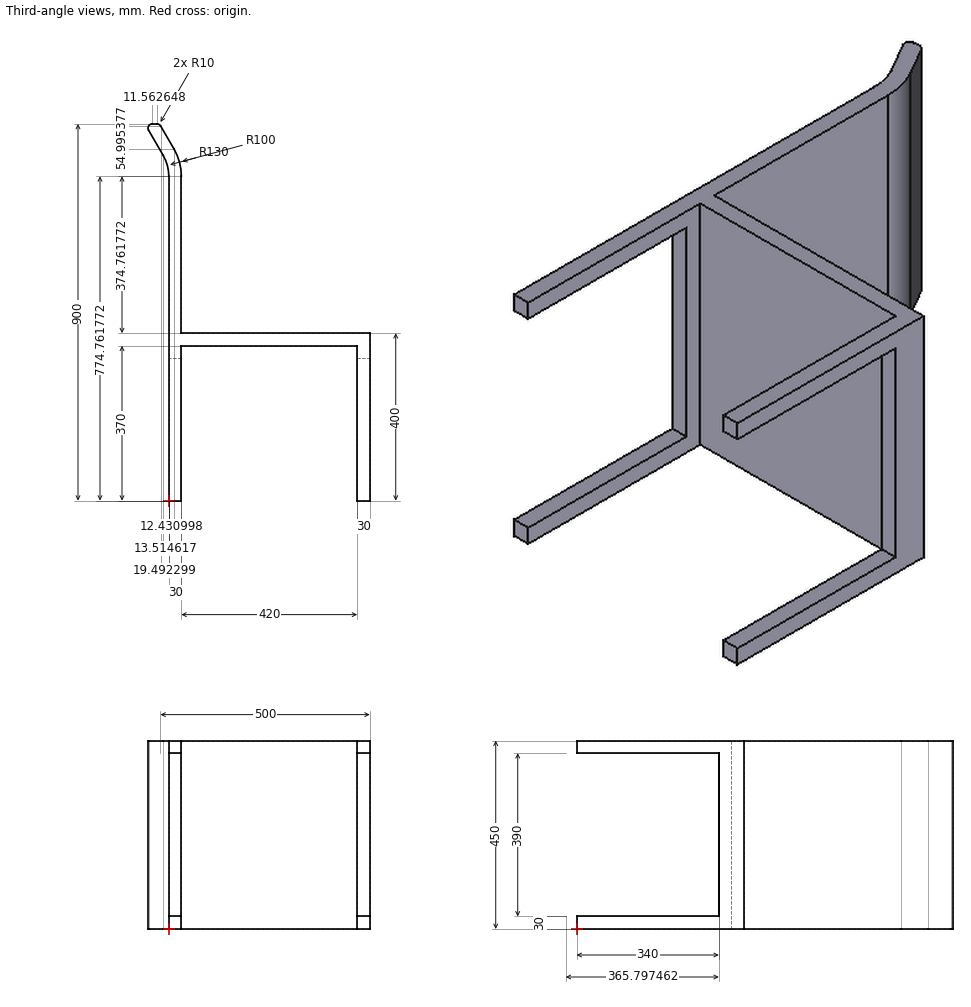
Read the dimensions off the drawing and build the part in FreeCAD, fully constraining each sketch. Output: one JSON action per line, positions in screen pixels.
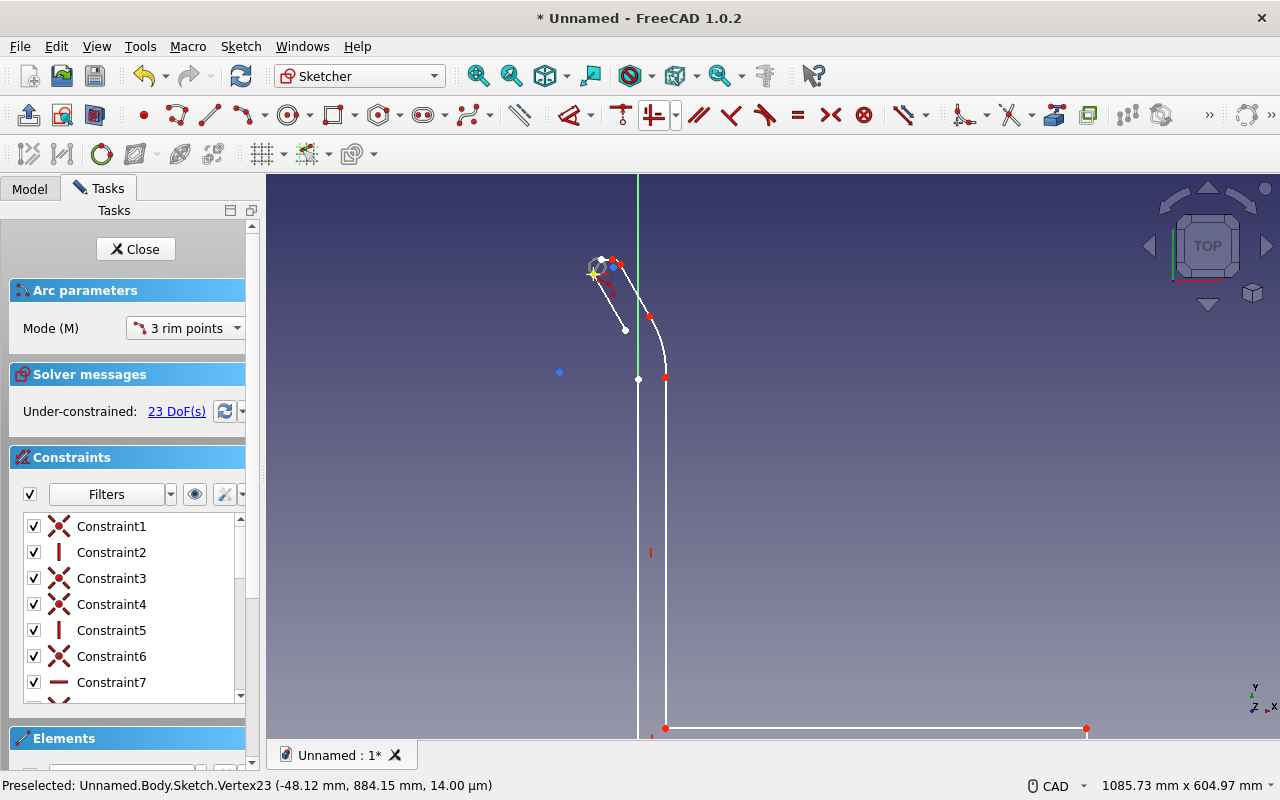
{"action": "scroll", "coordinate": [593, 264], "scroll_direction": "up", "scroll_amount": 7}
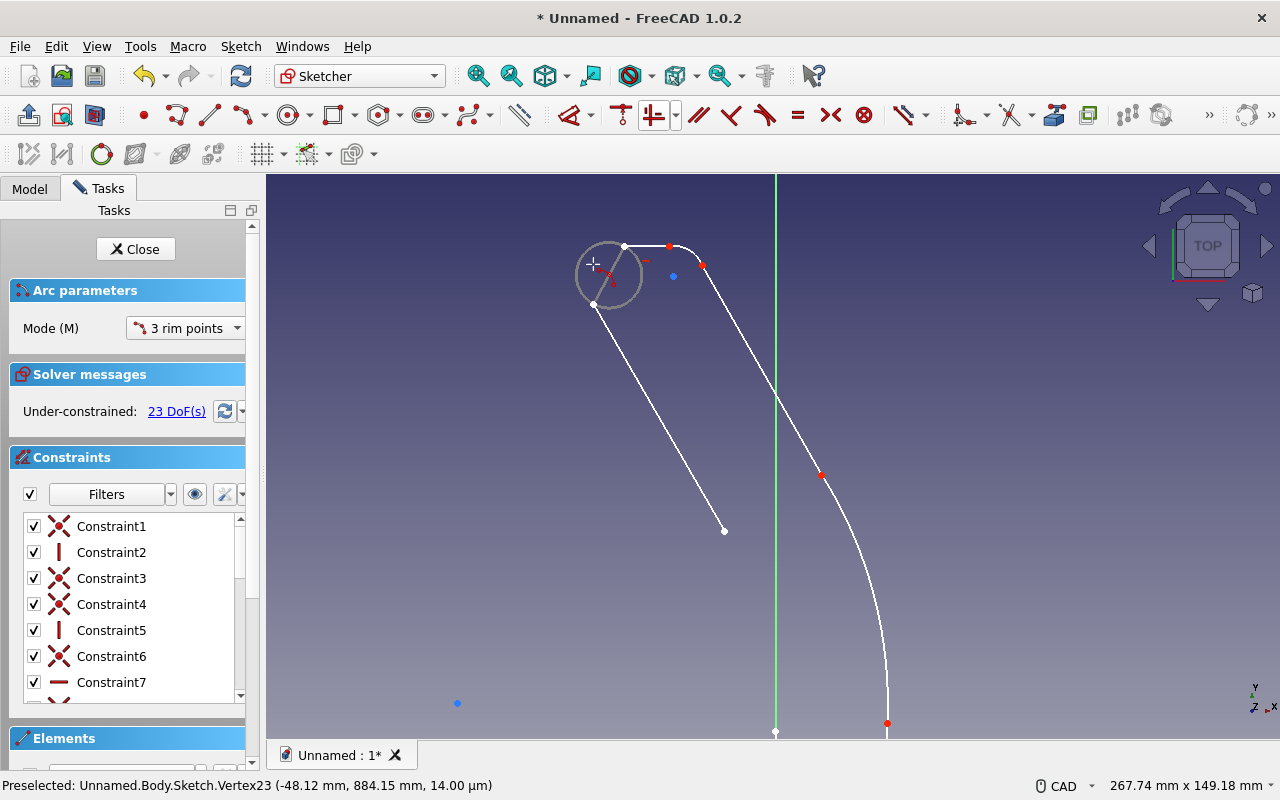
{"action": "left_click", "coordinate": [593, 263]}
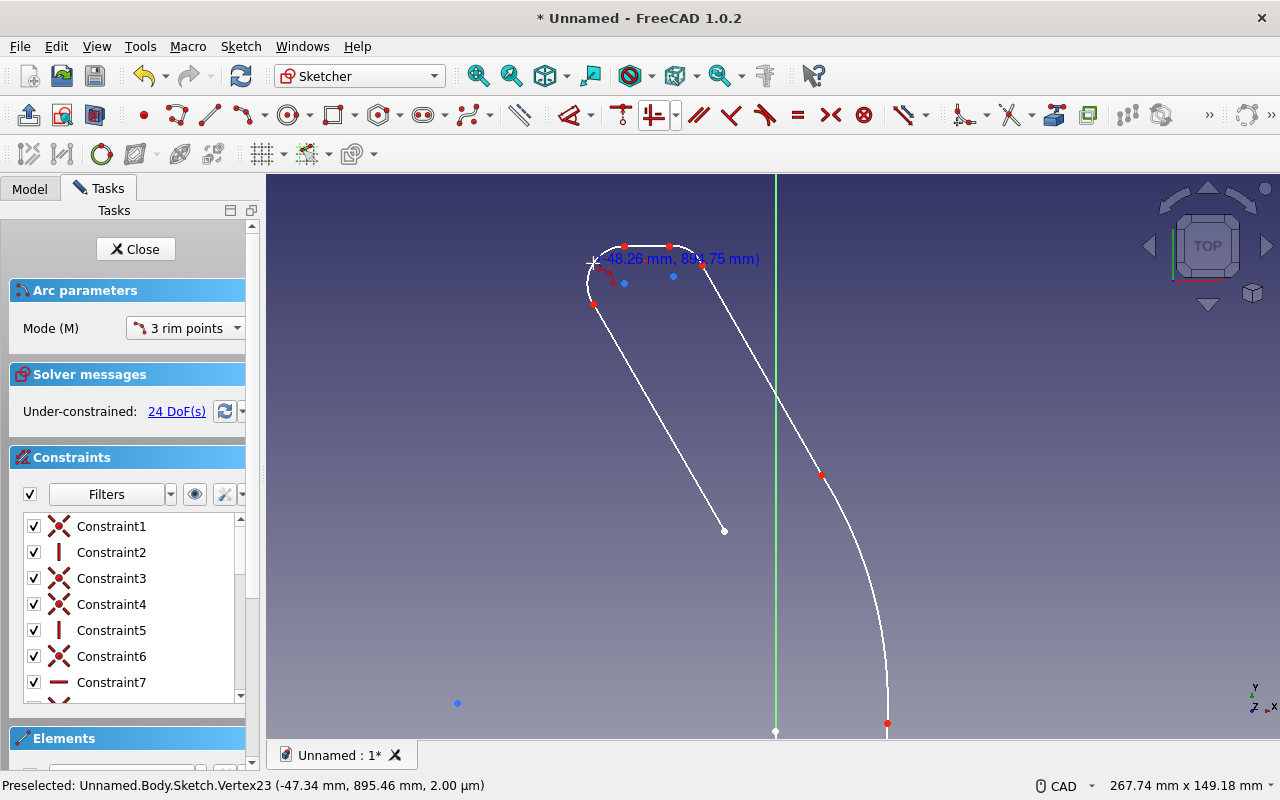
{"action": "scroll", "coordinate": [594, 271], "scroll_direction": "down", "scroll_amount": 11}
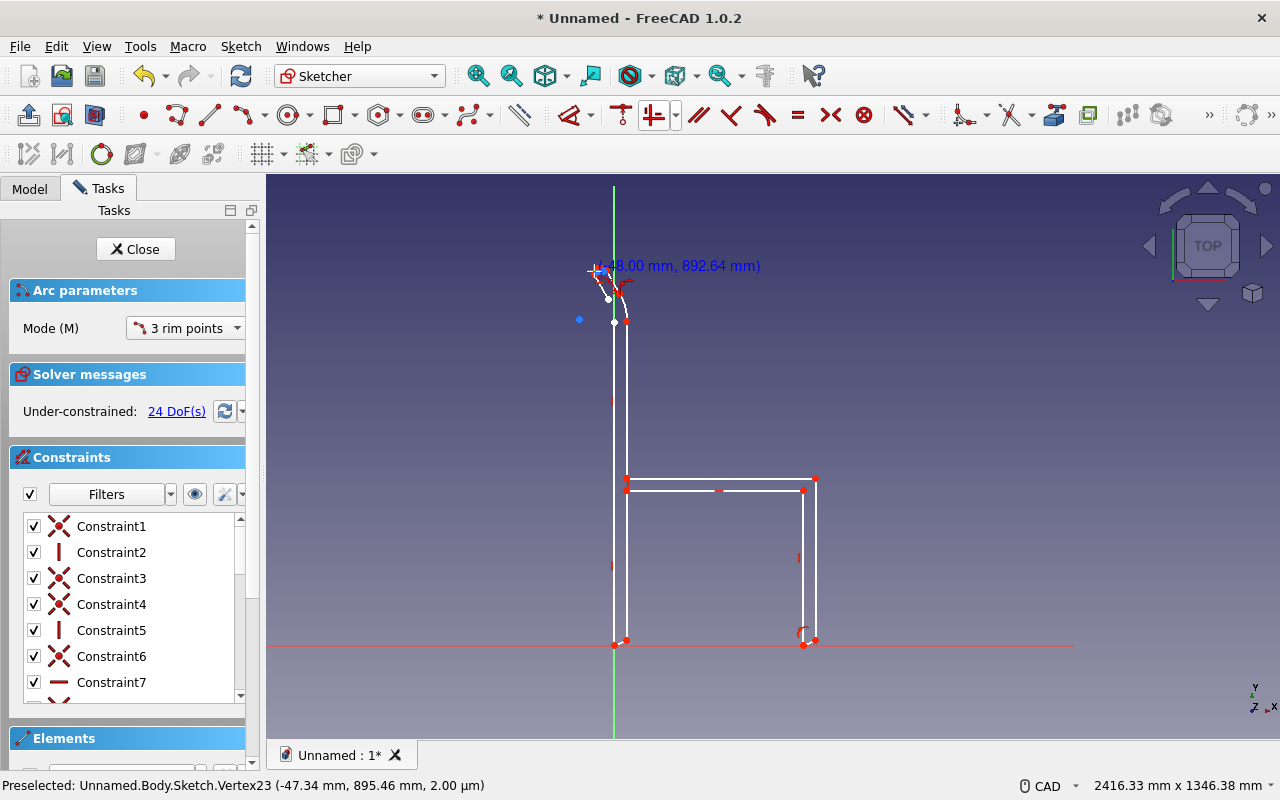
{"action": "scroll", "coordinate": [609, 300], "scroll_direction": "up", "scroll_amount": 6}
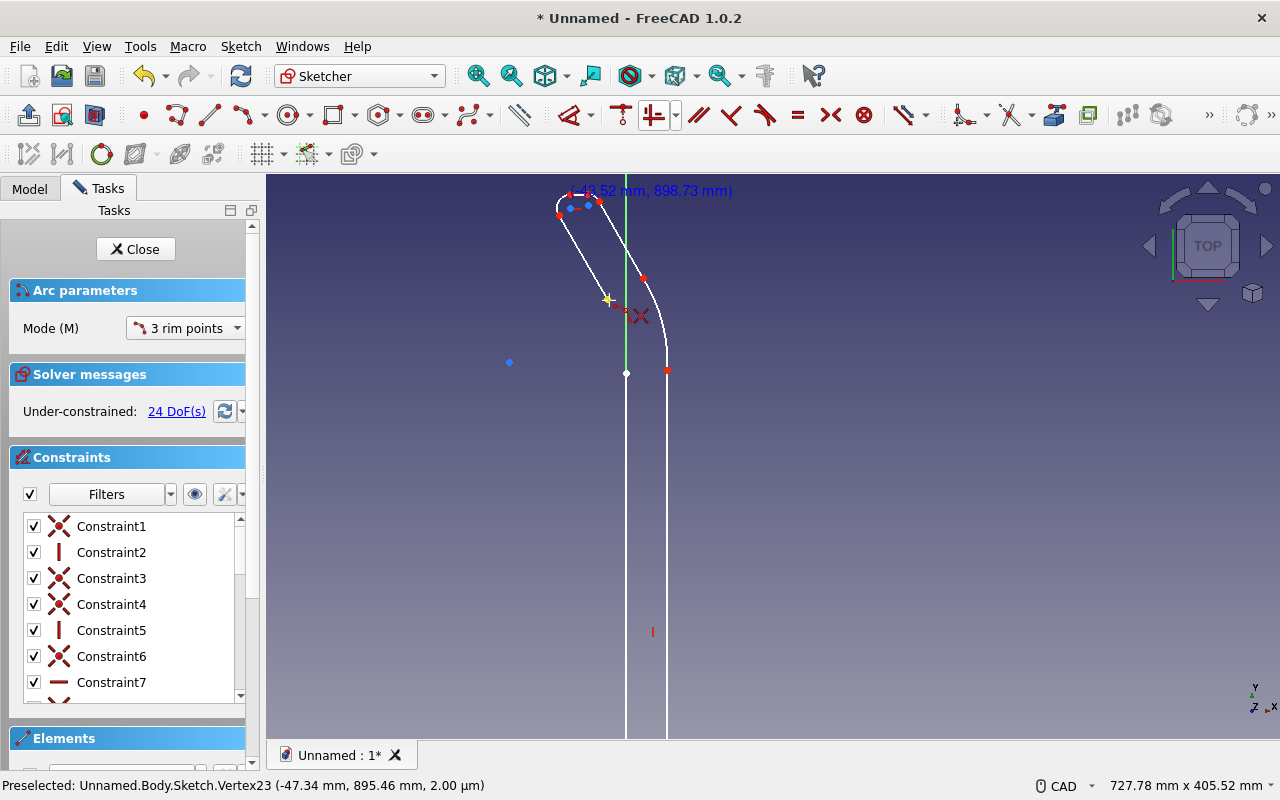
{"action": "left_click", "coordinate": [608, 299]}
{"action": "left_click", "coordinate": [626, 373]}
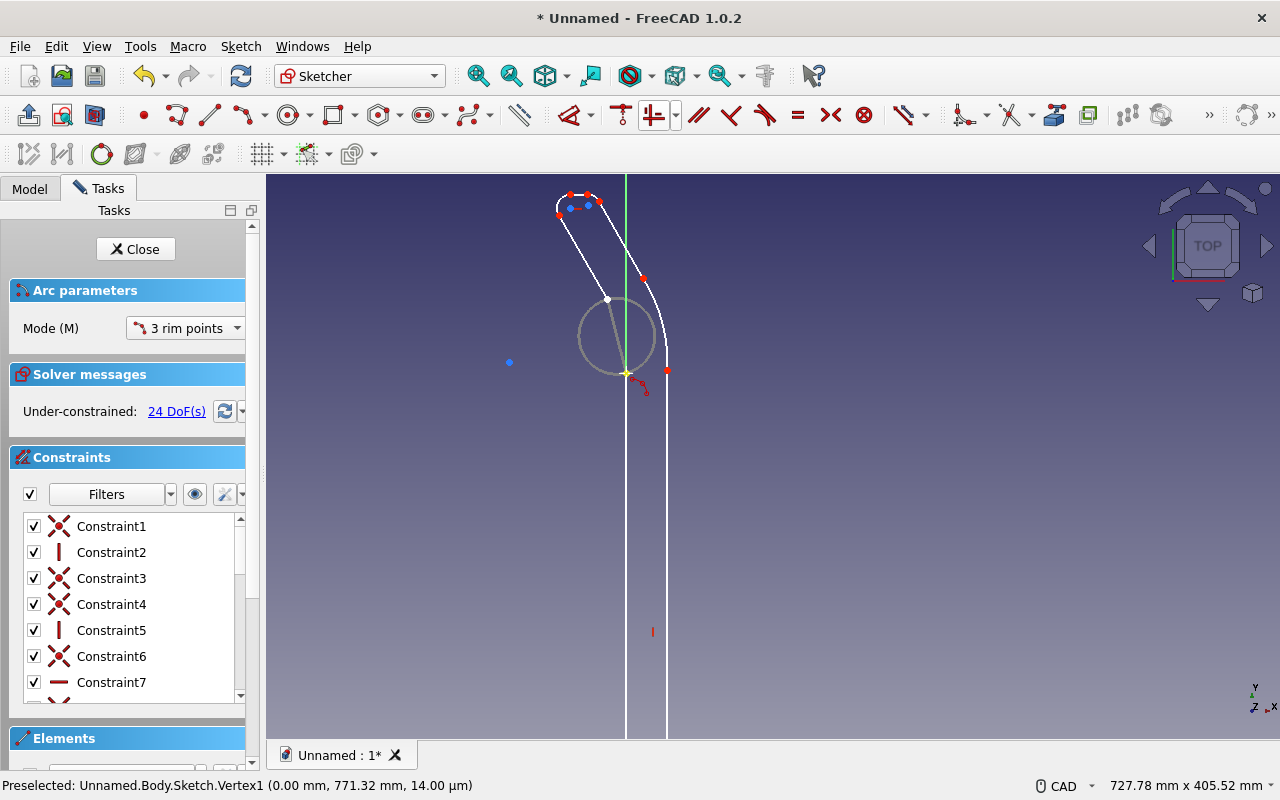
{"action": "scroll", "coordinate": [621, 332], "scroll_direction": "up", "scroll_amount": 6}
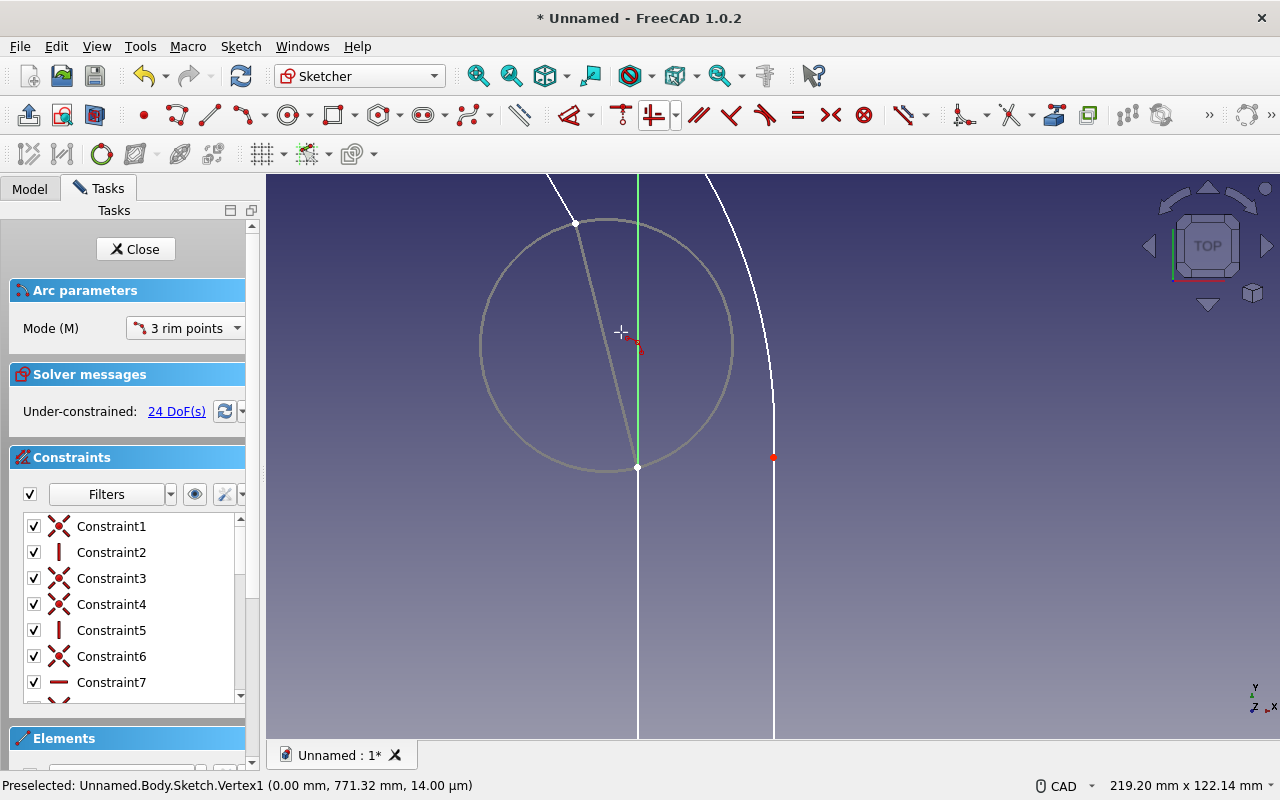
{"action": "left_click", "coordinate": [622, 332]}
{"action": "key", "text": "Escape"}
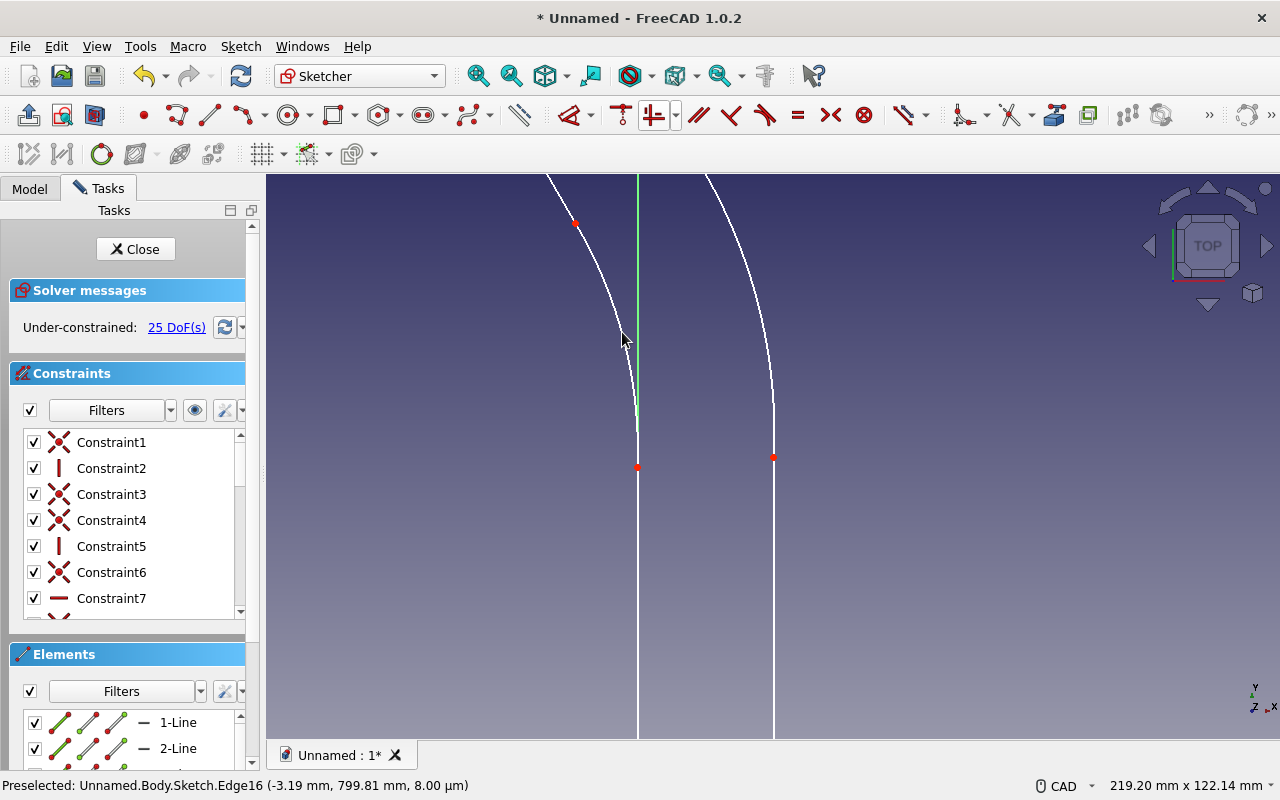
{"action": "scroll", "coordinate": [612, 307], "scroll_direction": "down", "scroll_amount": 12}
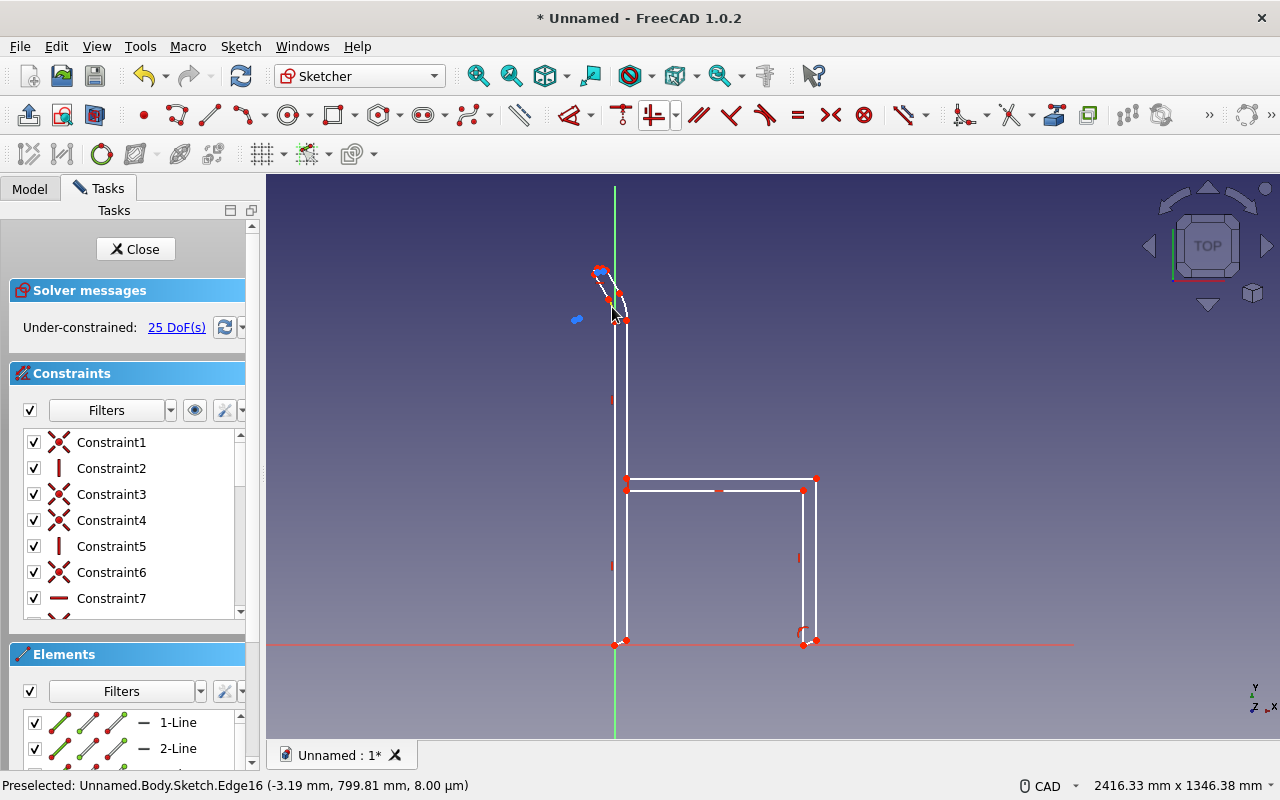
{"action": "scroll", "coordinate": [616, 286], "scroll_direction": "up", "scroll_amount": 13}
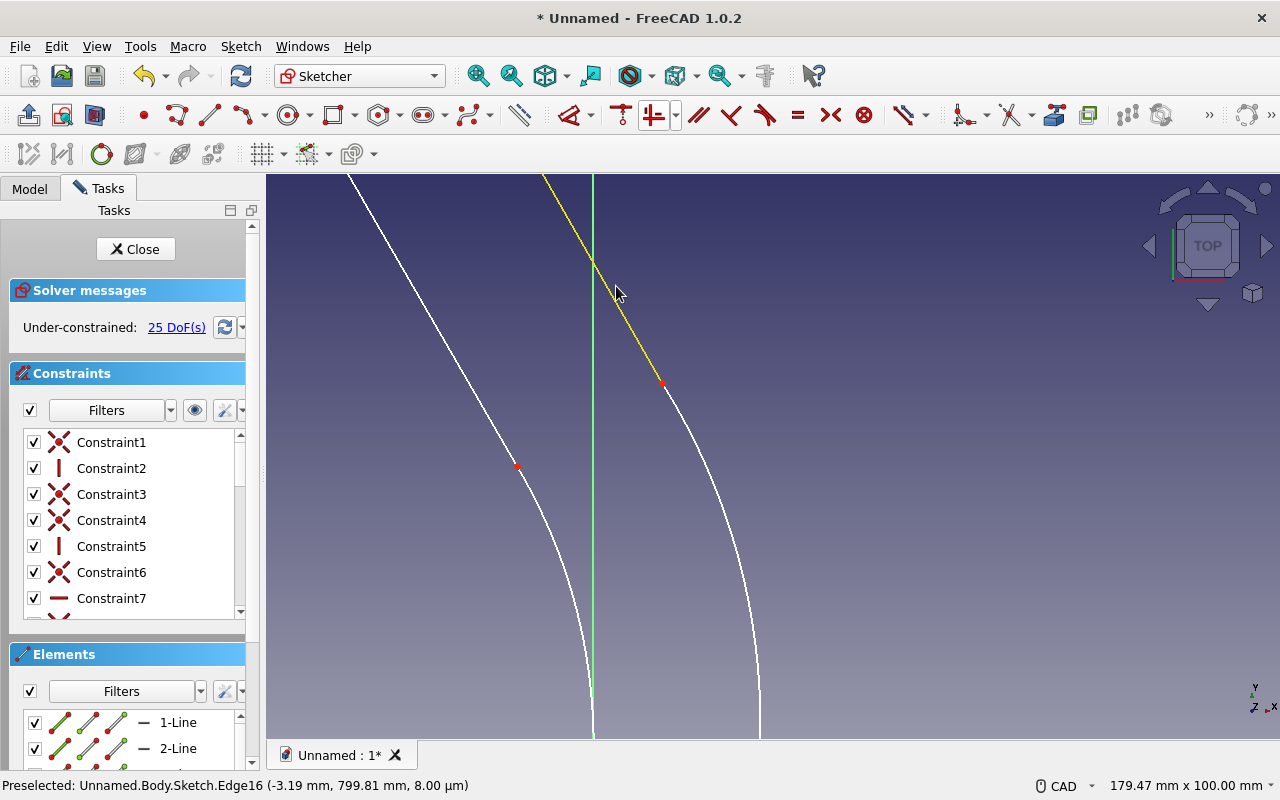
{"action": "left_click", "coordinate": [609, 290]}